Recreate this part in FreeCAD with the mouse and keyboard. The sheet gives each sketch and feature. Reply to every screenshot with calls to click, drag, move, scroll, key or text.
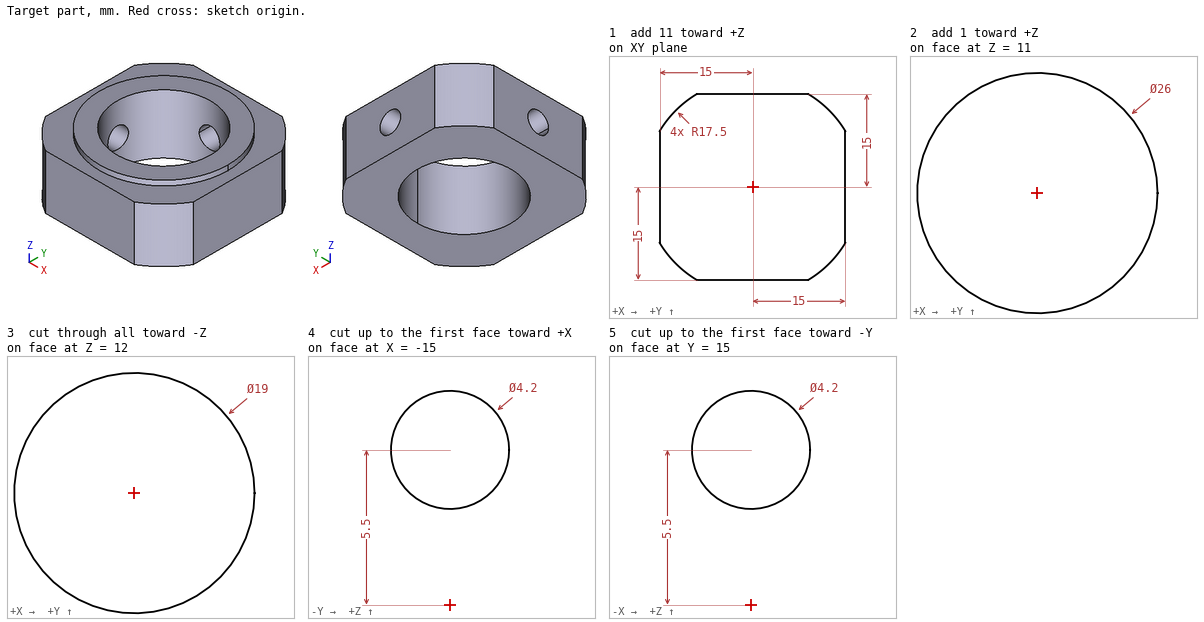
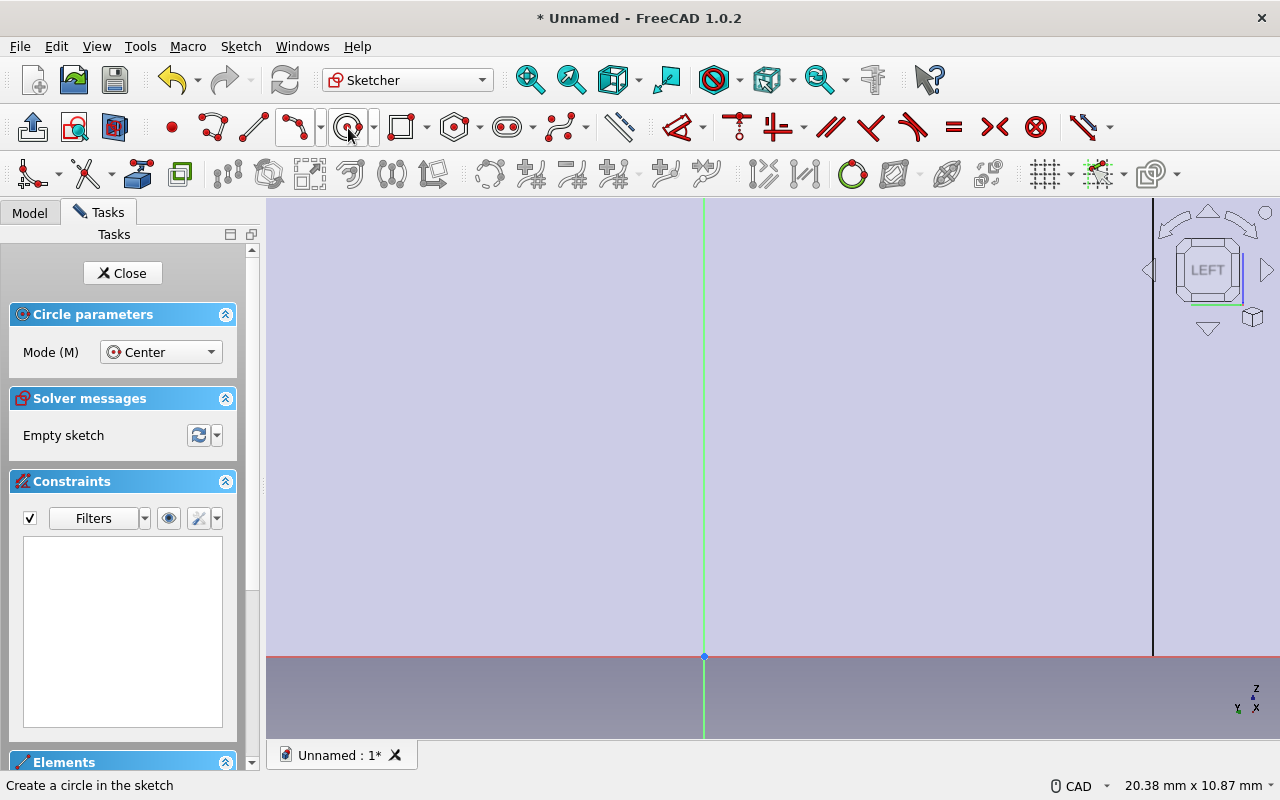
click(704, 383)
click(778, 309)
key(Escape)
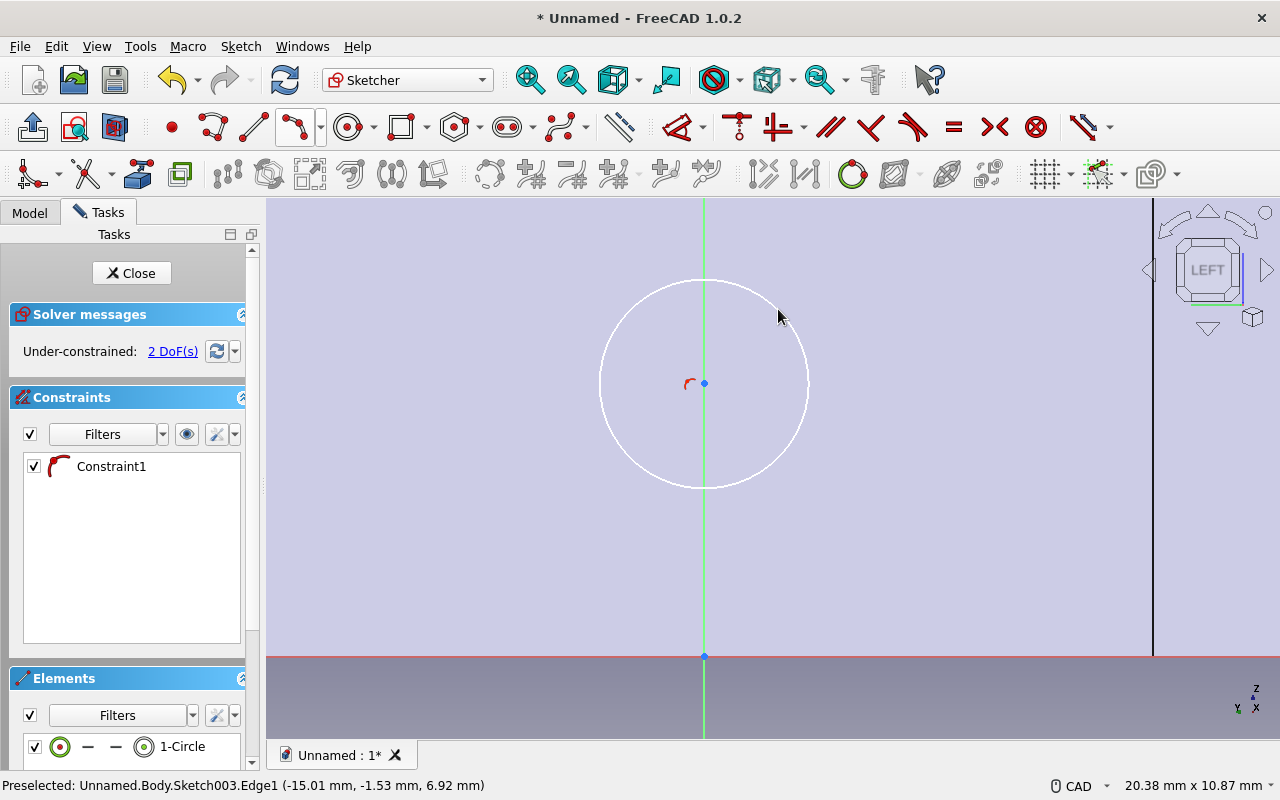
click(676, 128)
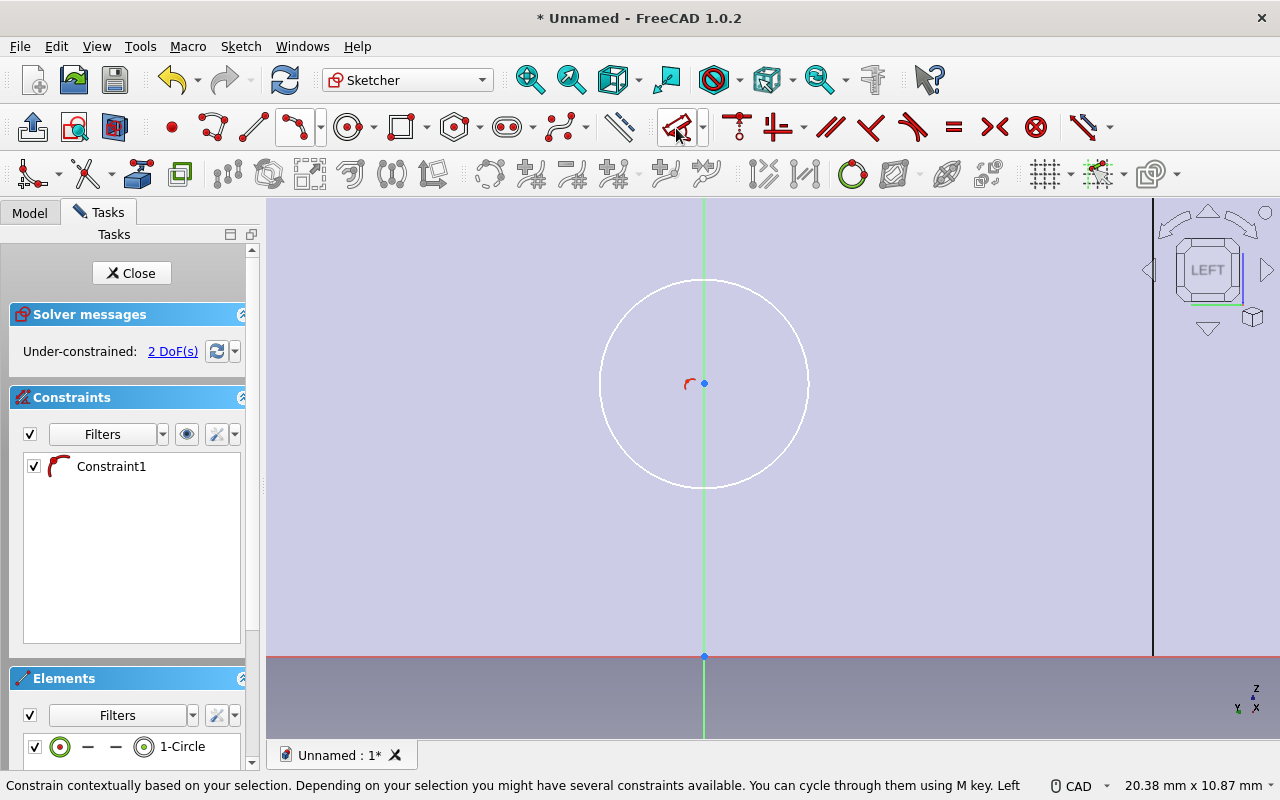
click(778, 310)
click(801, 287)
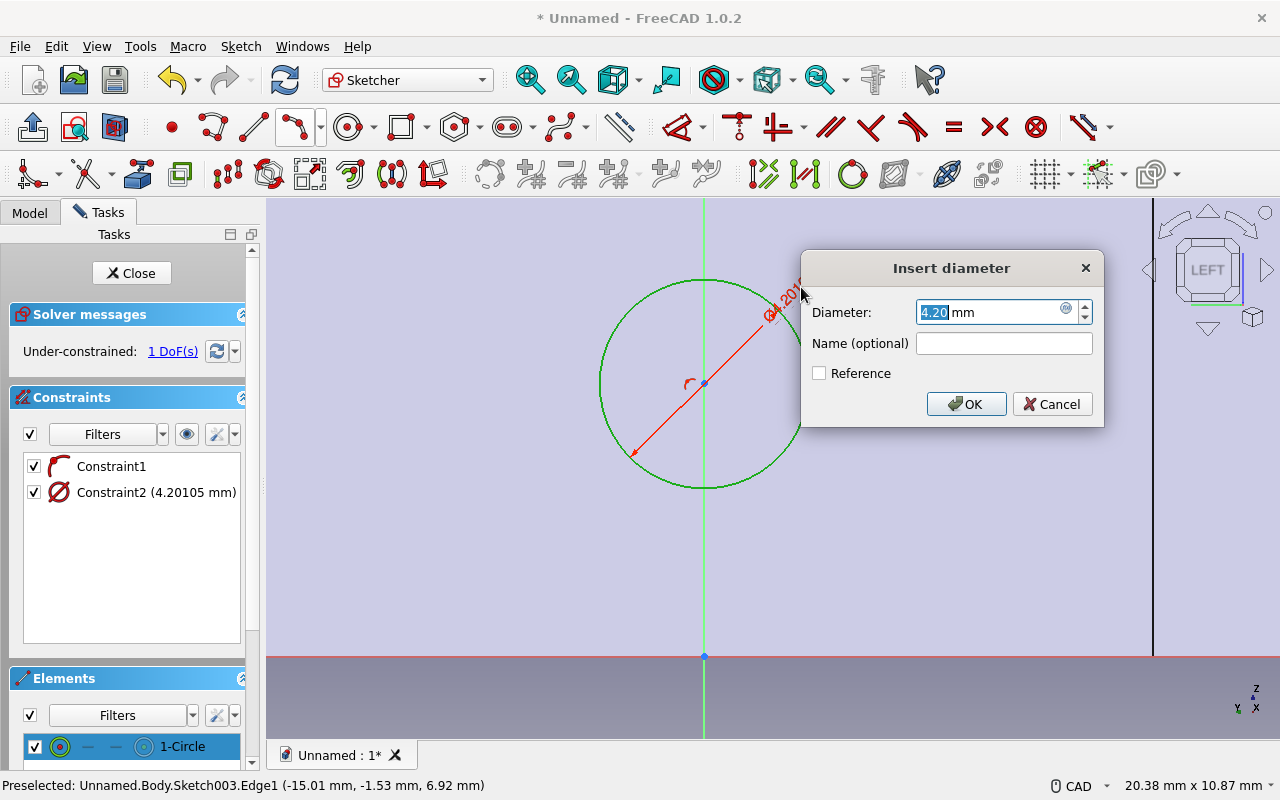
text(4.2)
key(Return)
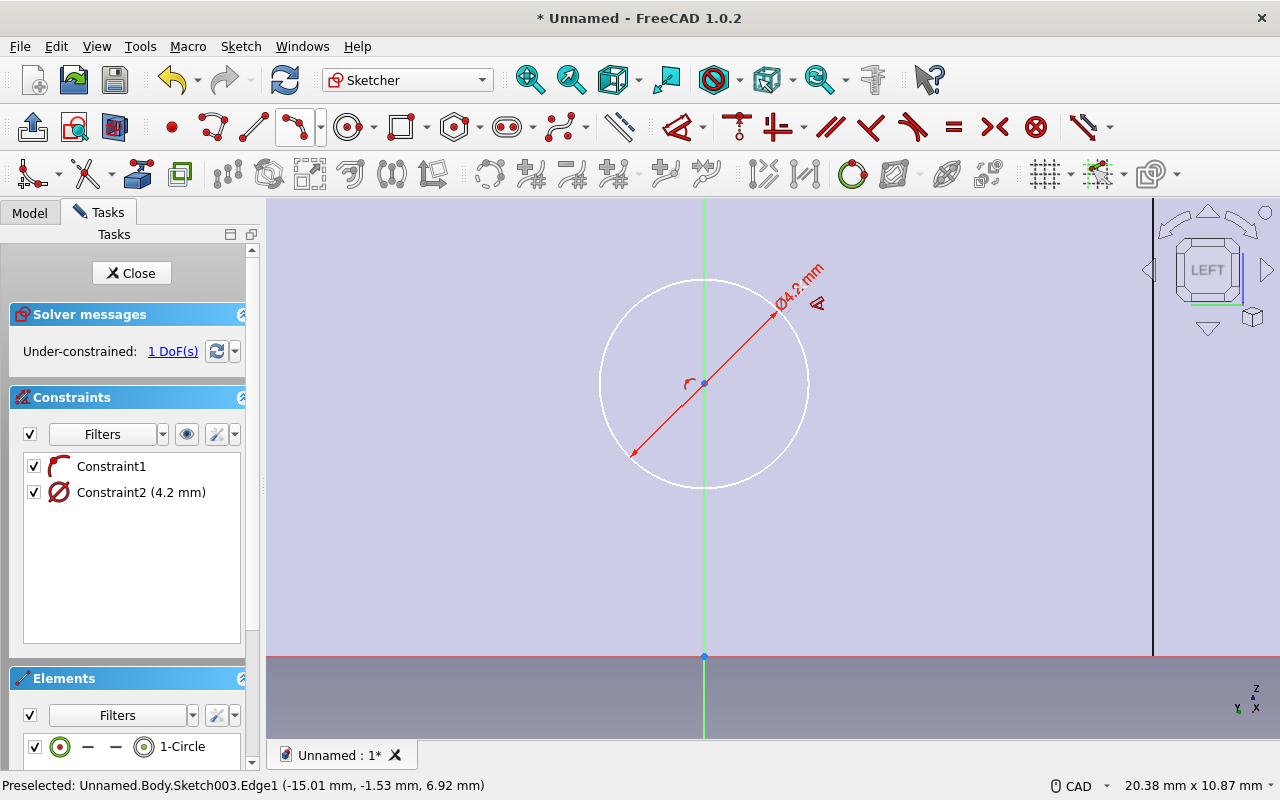
click(704, 384)
click(738, 520)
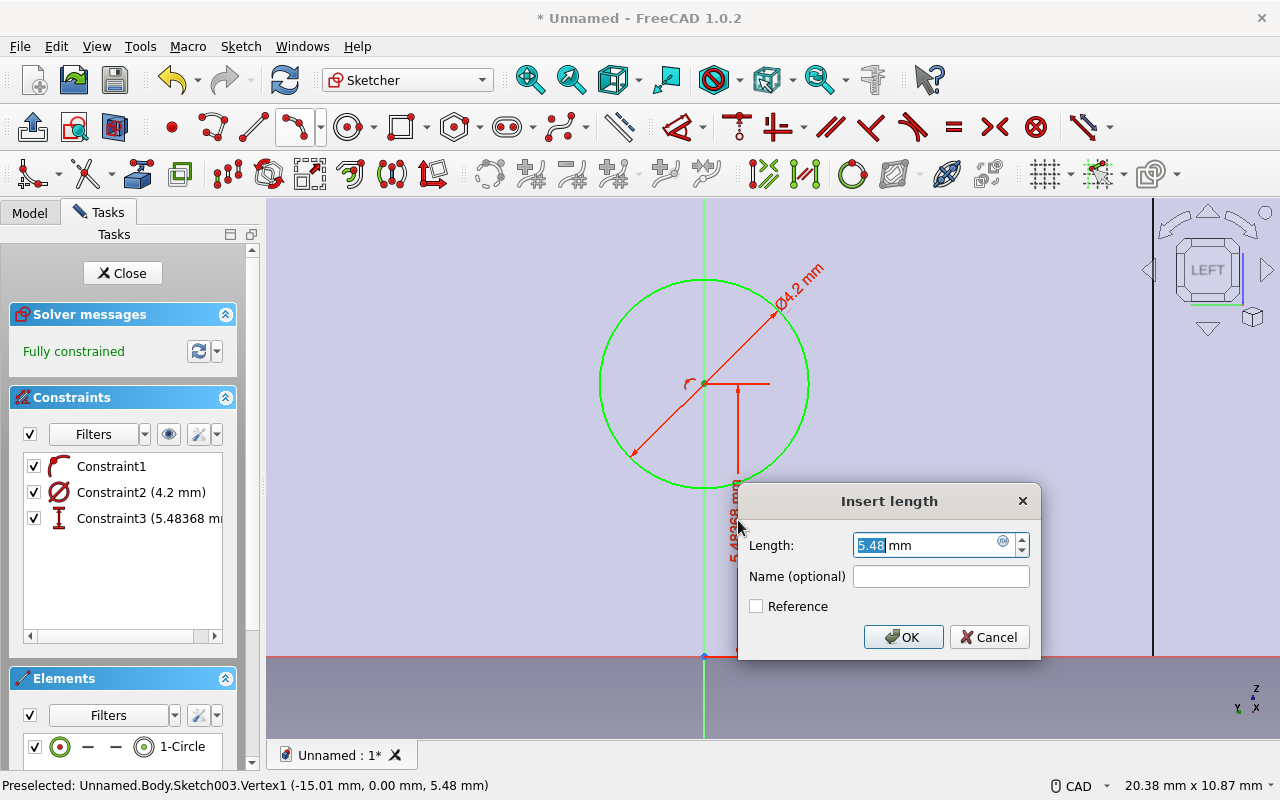
text(5.5)
key(Return)
key(Escape)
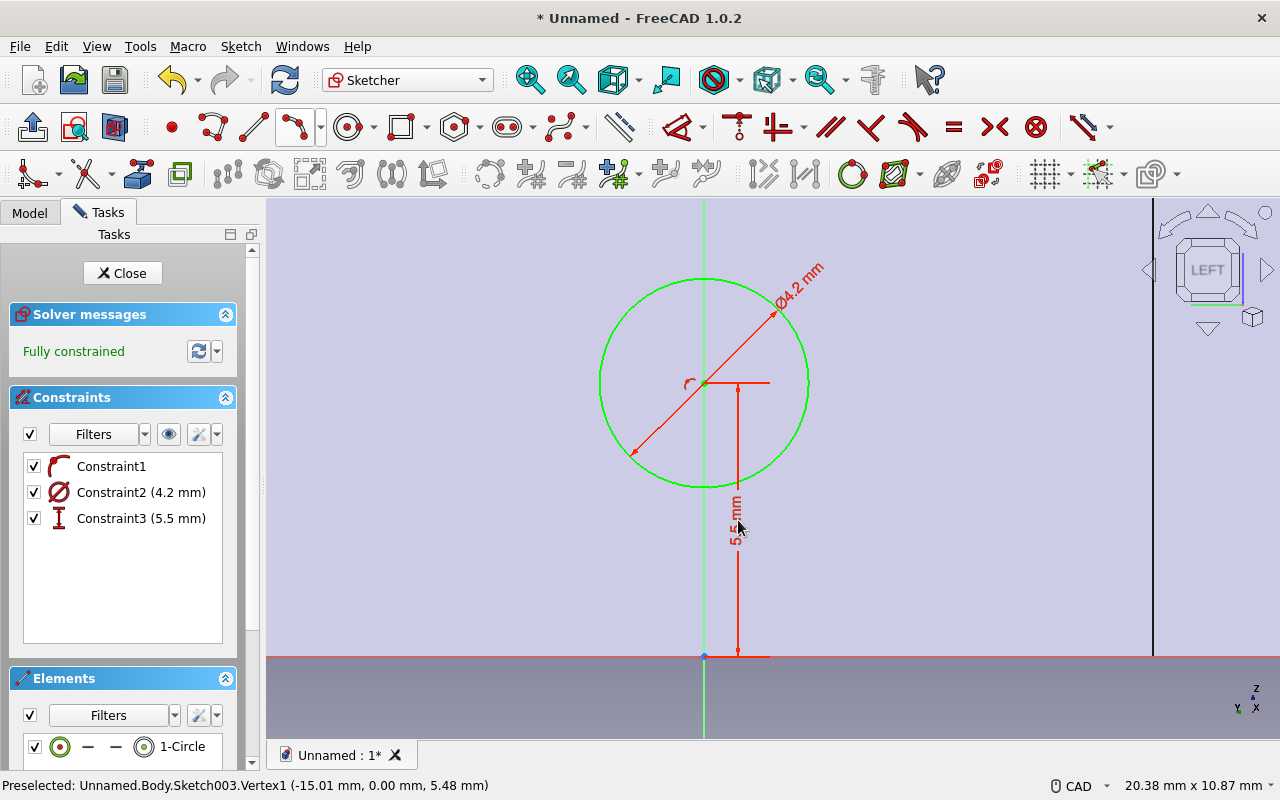
click(123, 273)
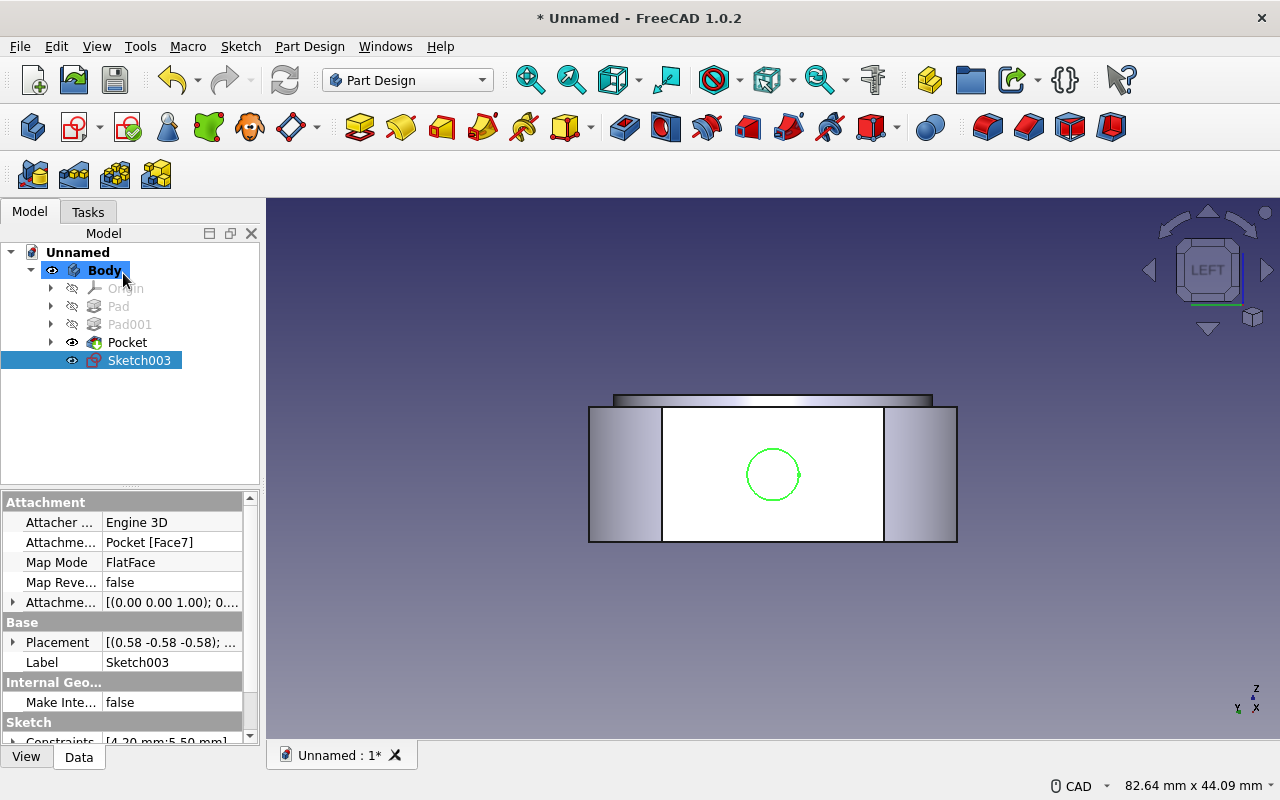
click(625, 128)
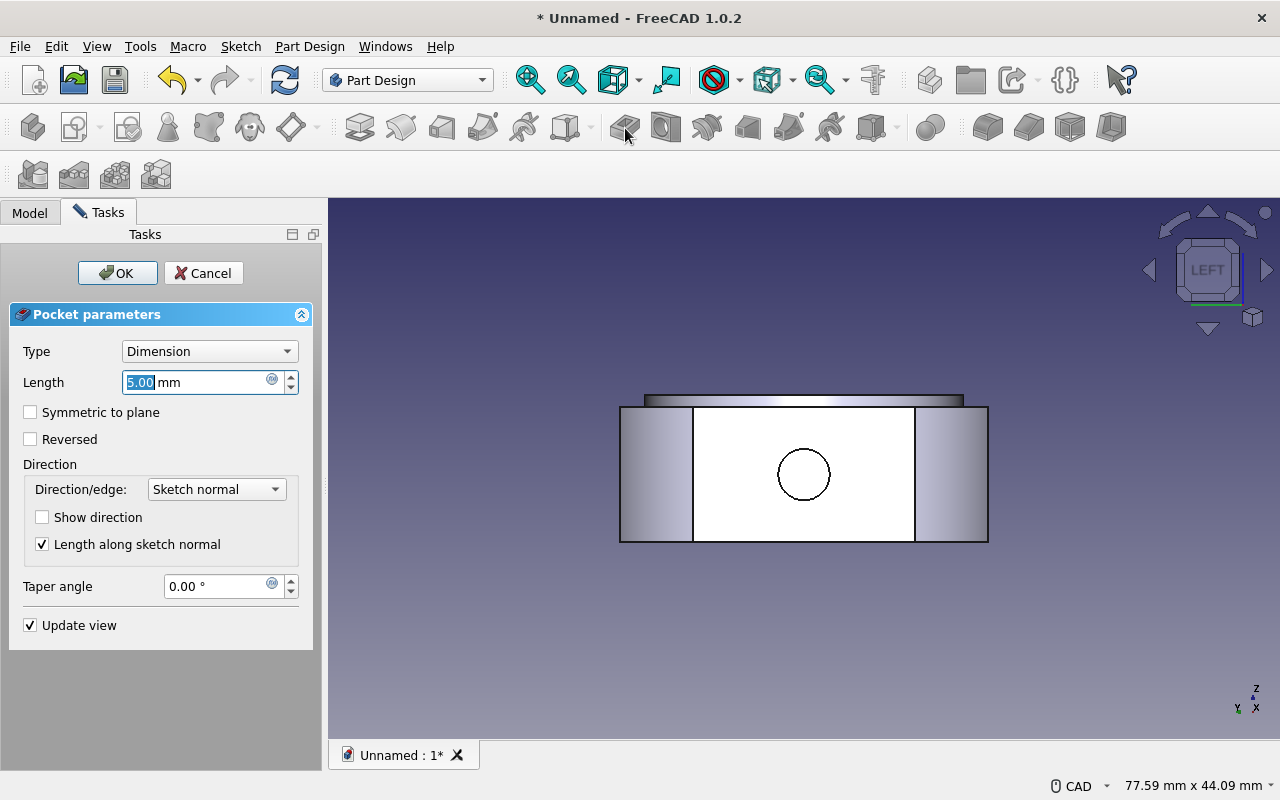
click(210, 352)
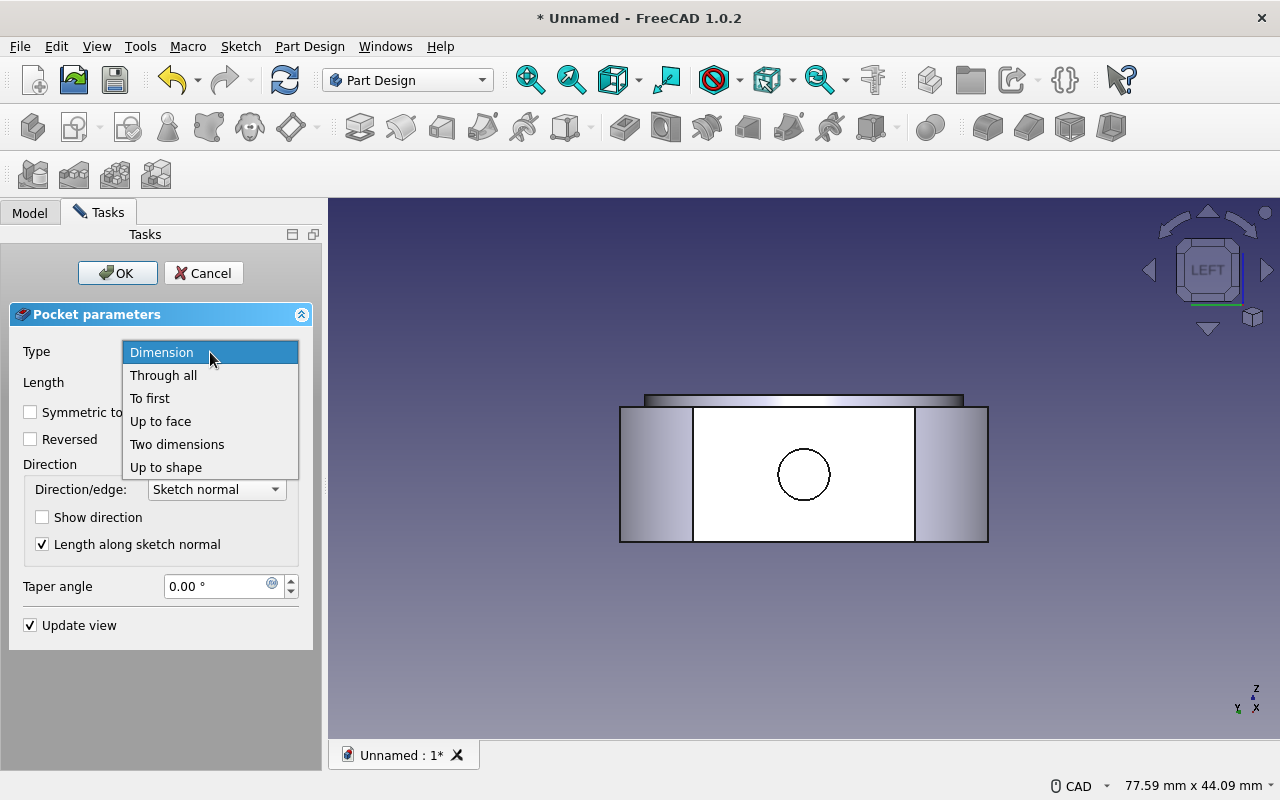
click(208, 398)